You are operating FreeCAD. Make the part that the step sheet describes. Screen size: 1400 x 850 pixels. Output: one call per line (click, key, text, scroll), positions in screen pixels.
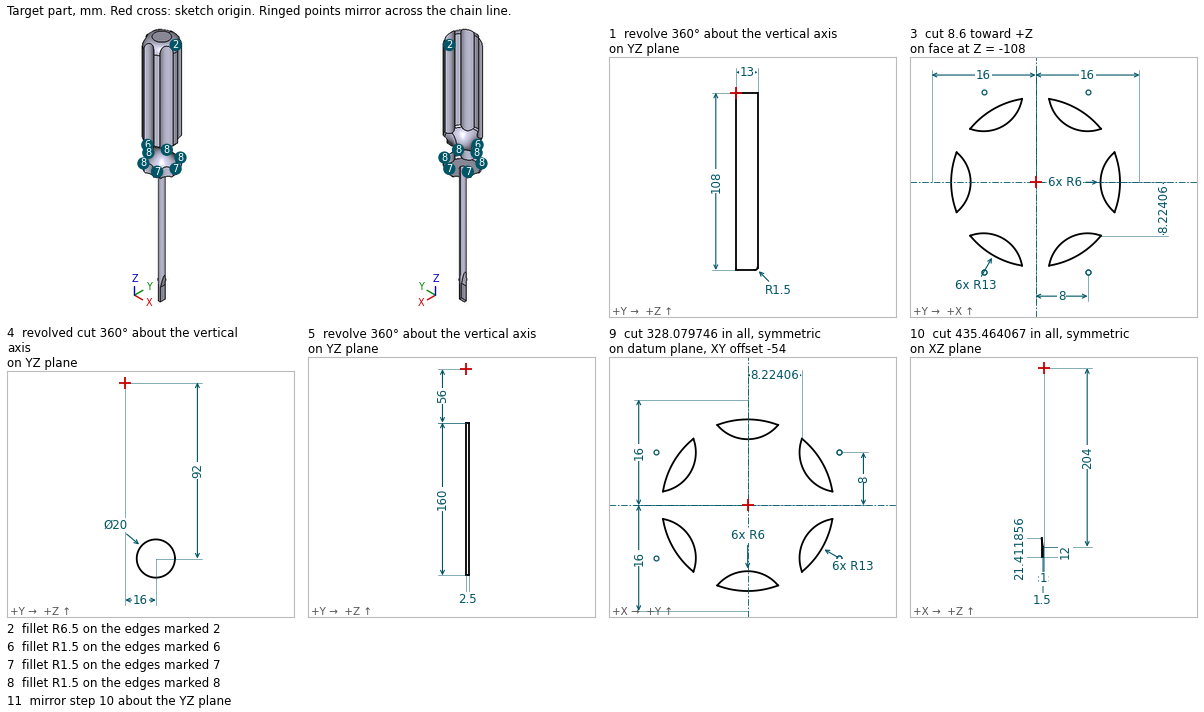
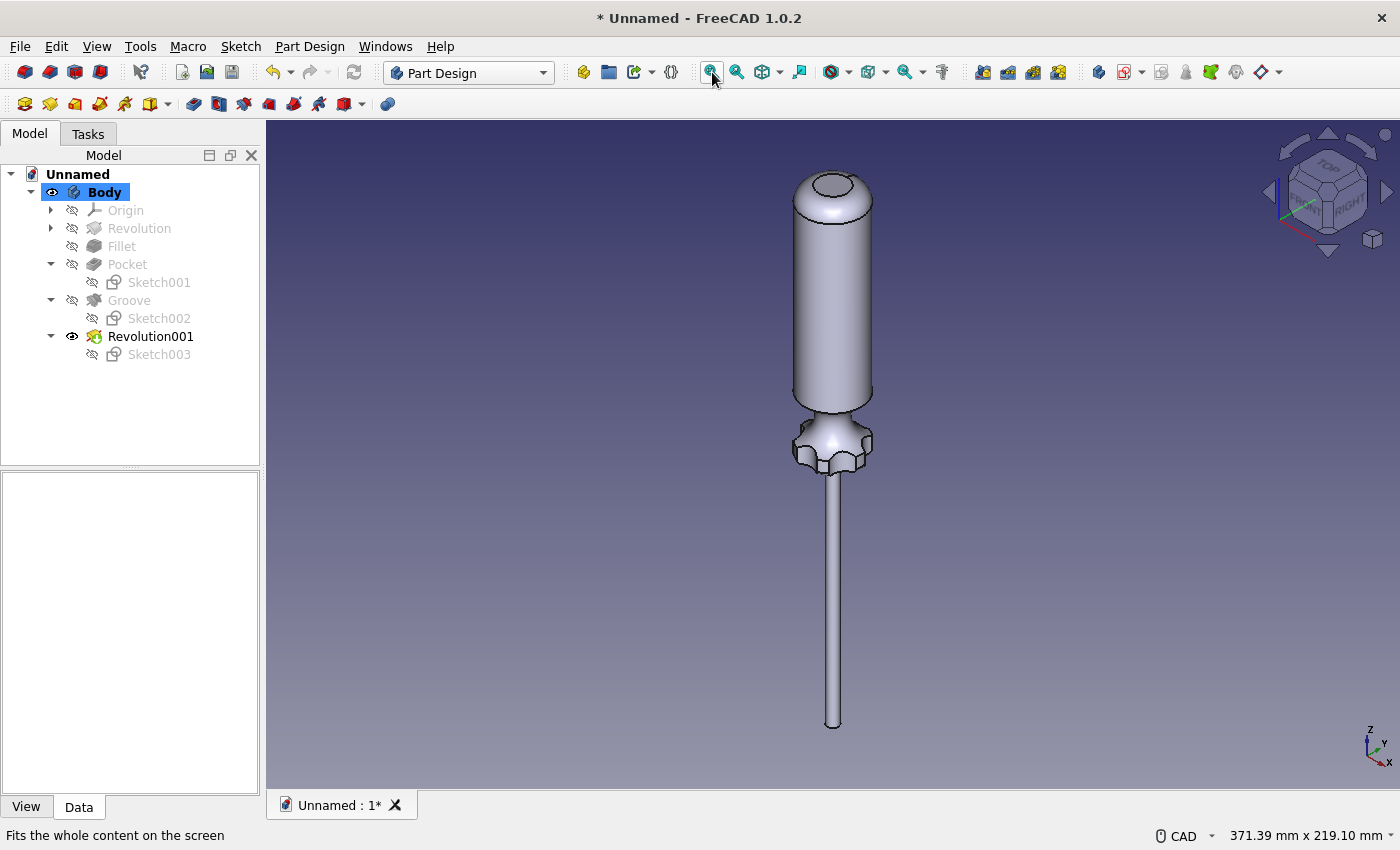
key(2)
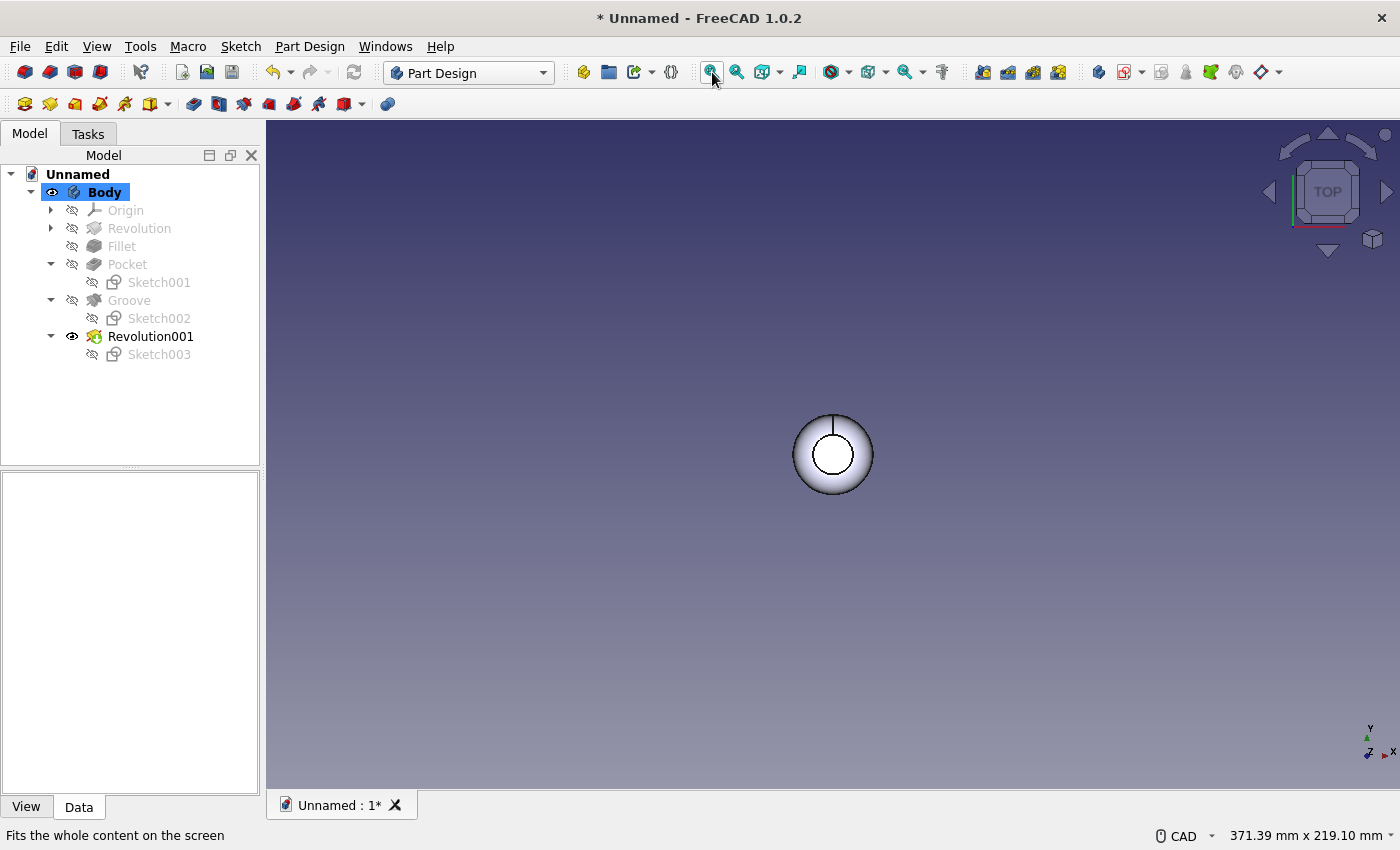
click(712, 72)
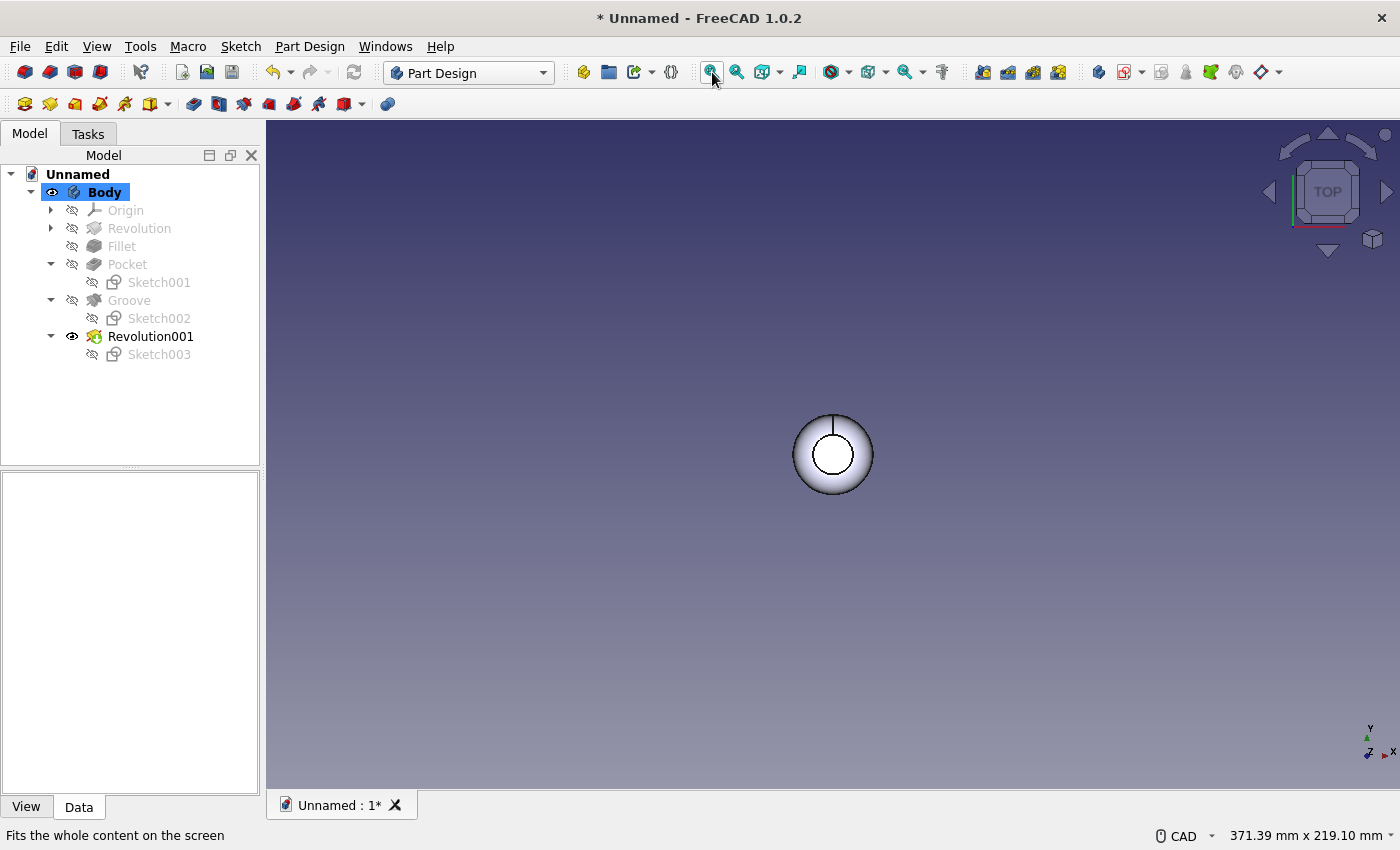
key(1)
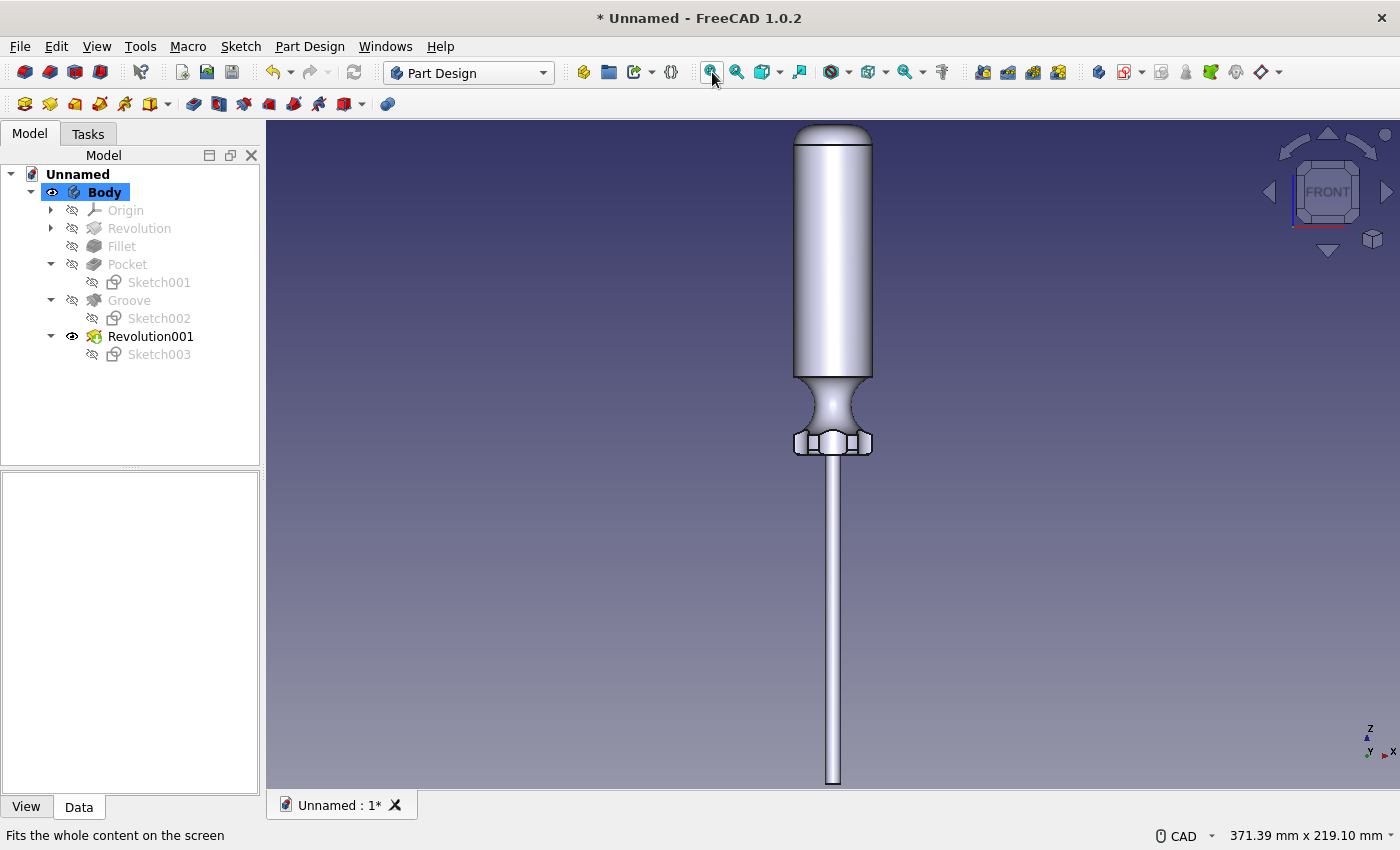
click(833, 376)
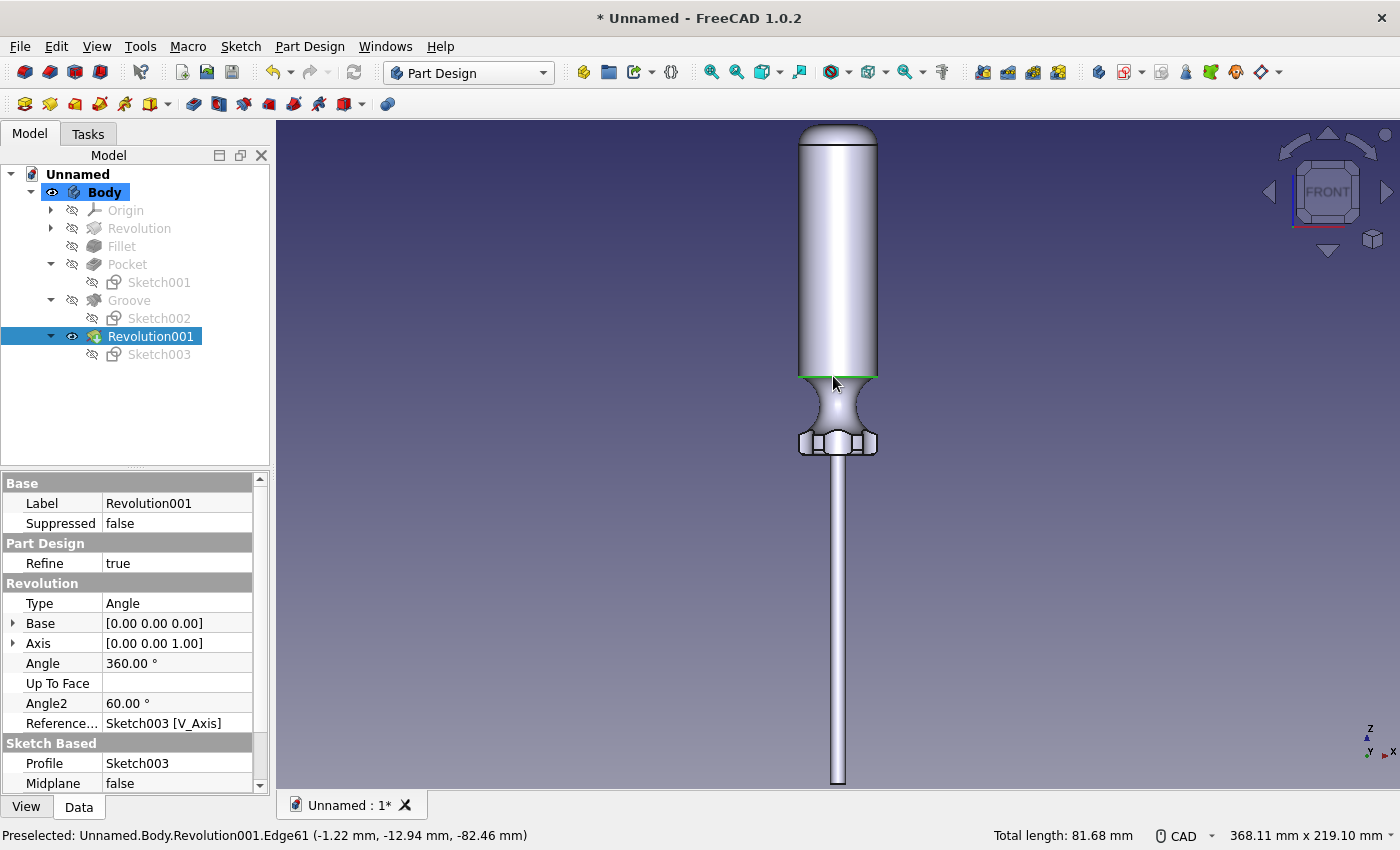
click(25, 72)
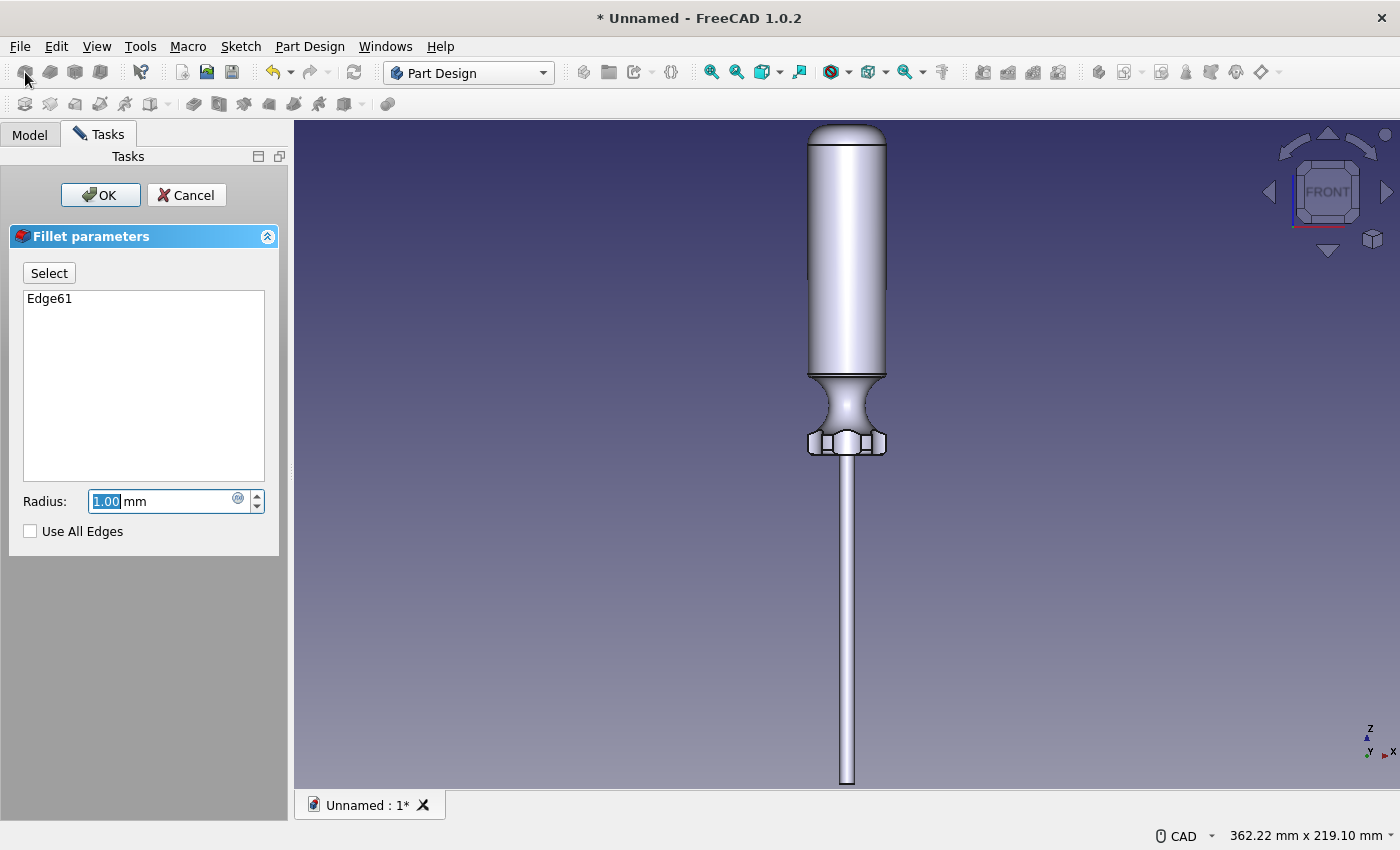
text(1.5)
key(Tab)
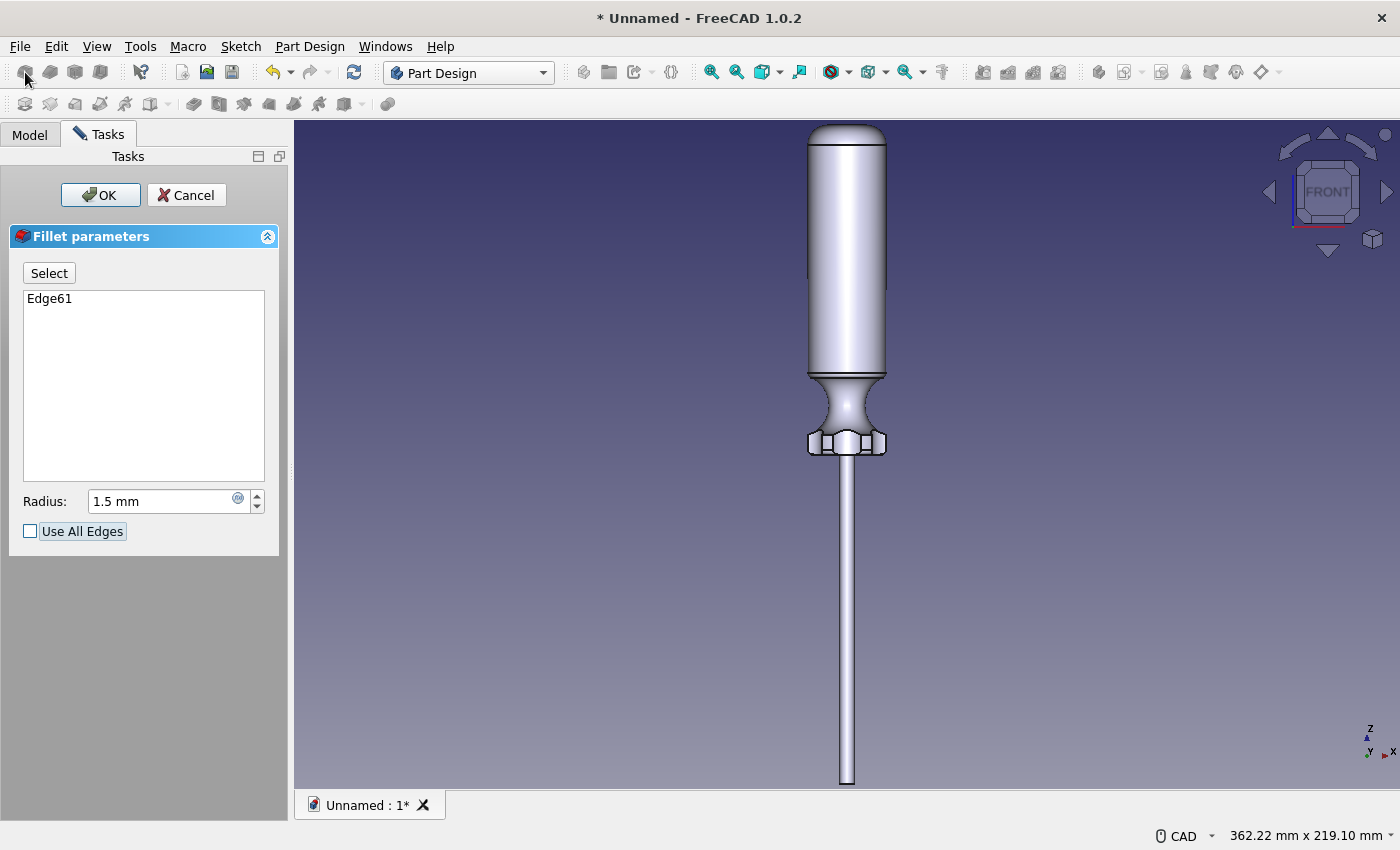
click(101, 195)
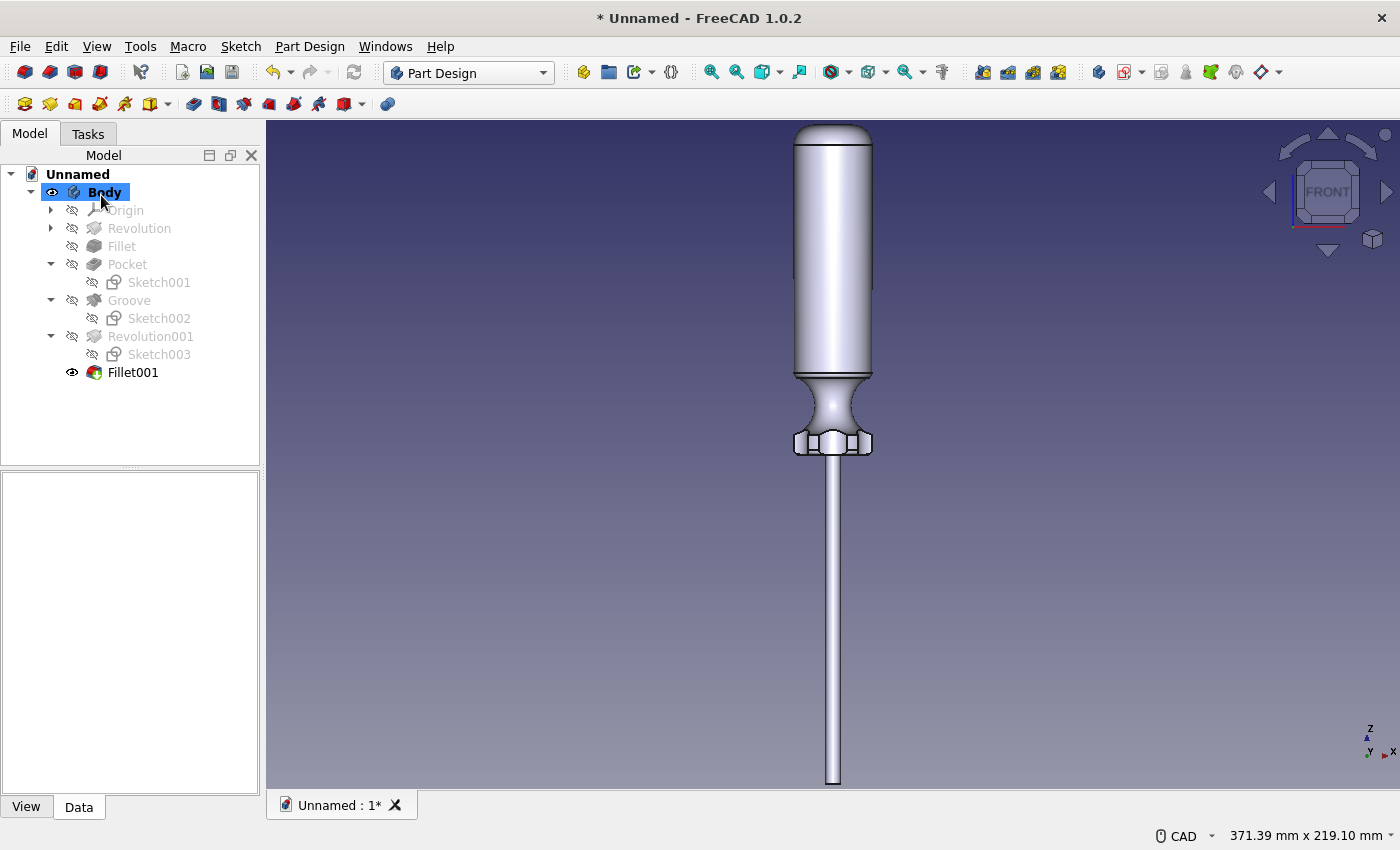
click(854, 434)